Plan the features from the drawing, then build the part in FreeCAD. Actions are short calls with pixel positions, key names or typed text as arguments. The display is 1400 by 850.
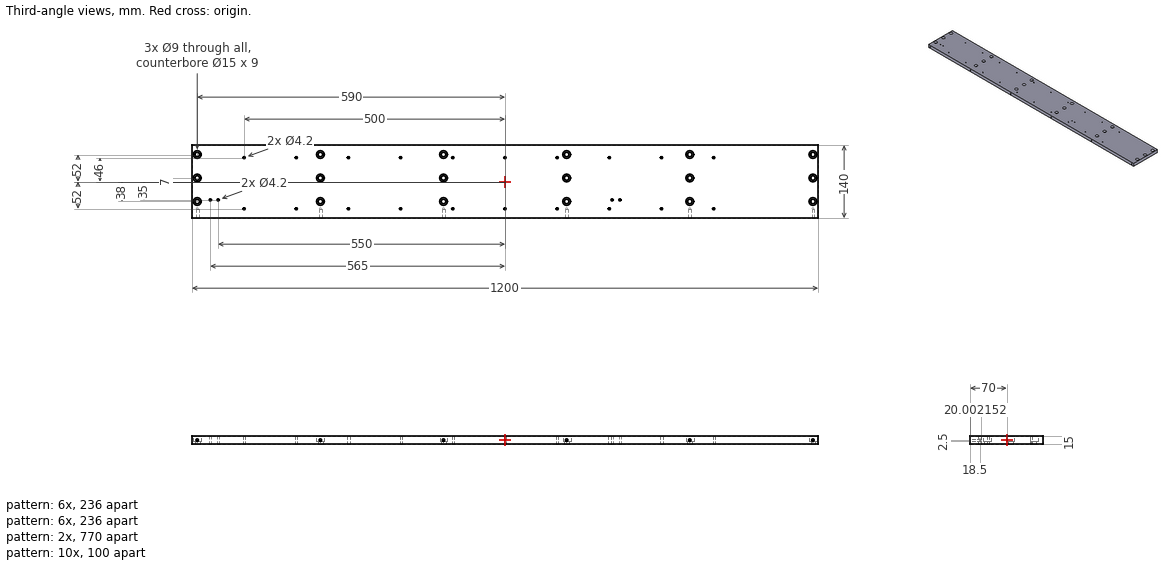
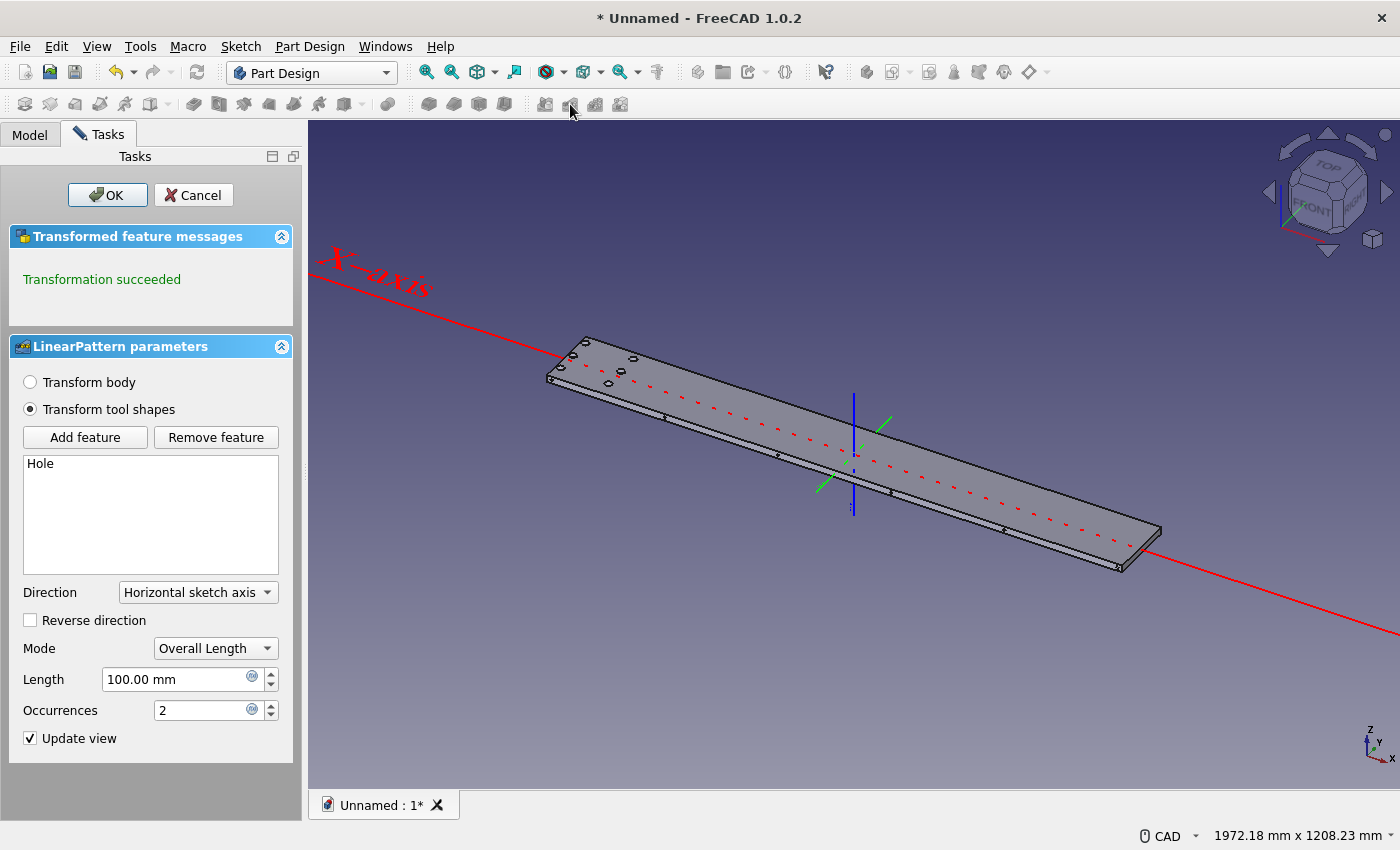
click(199, 592)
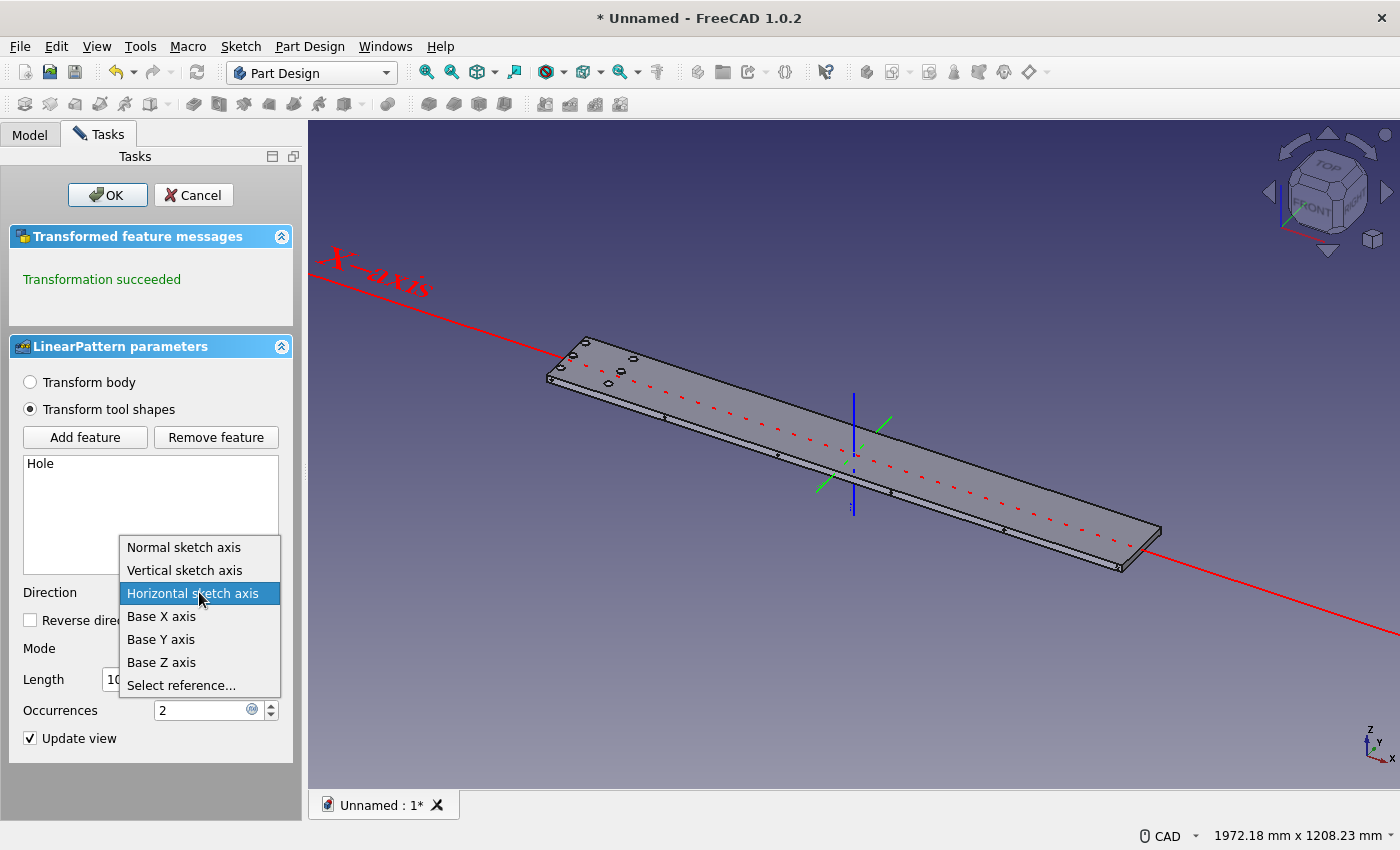
click(198, 616)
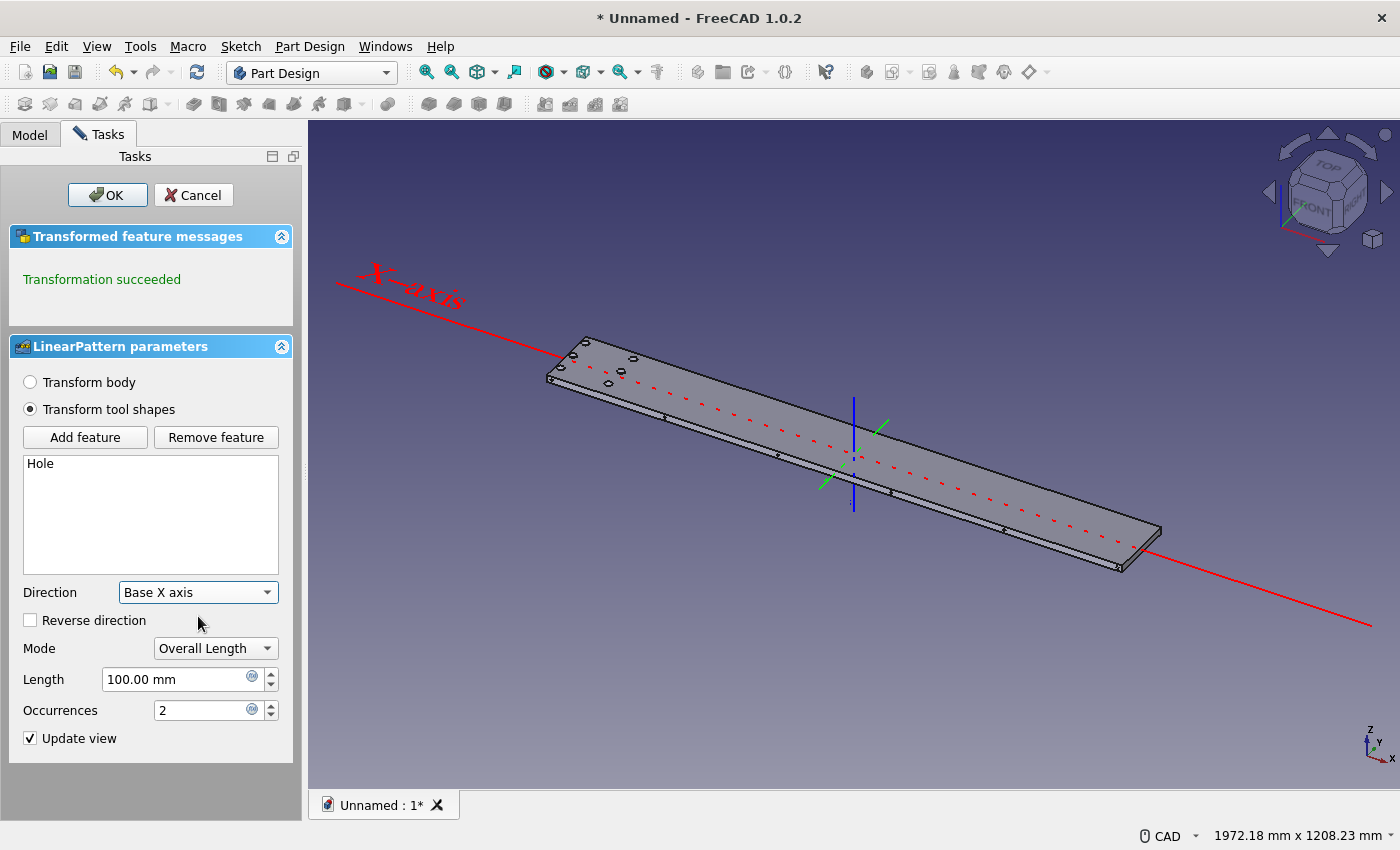
click(216, 648)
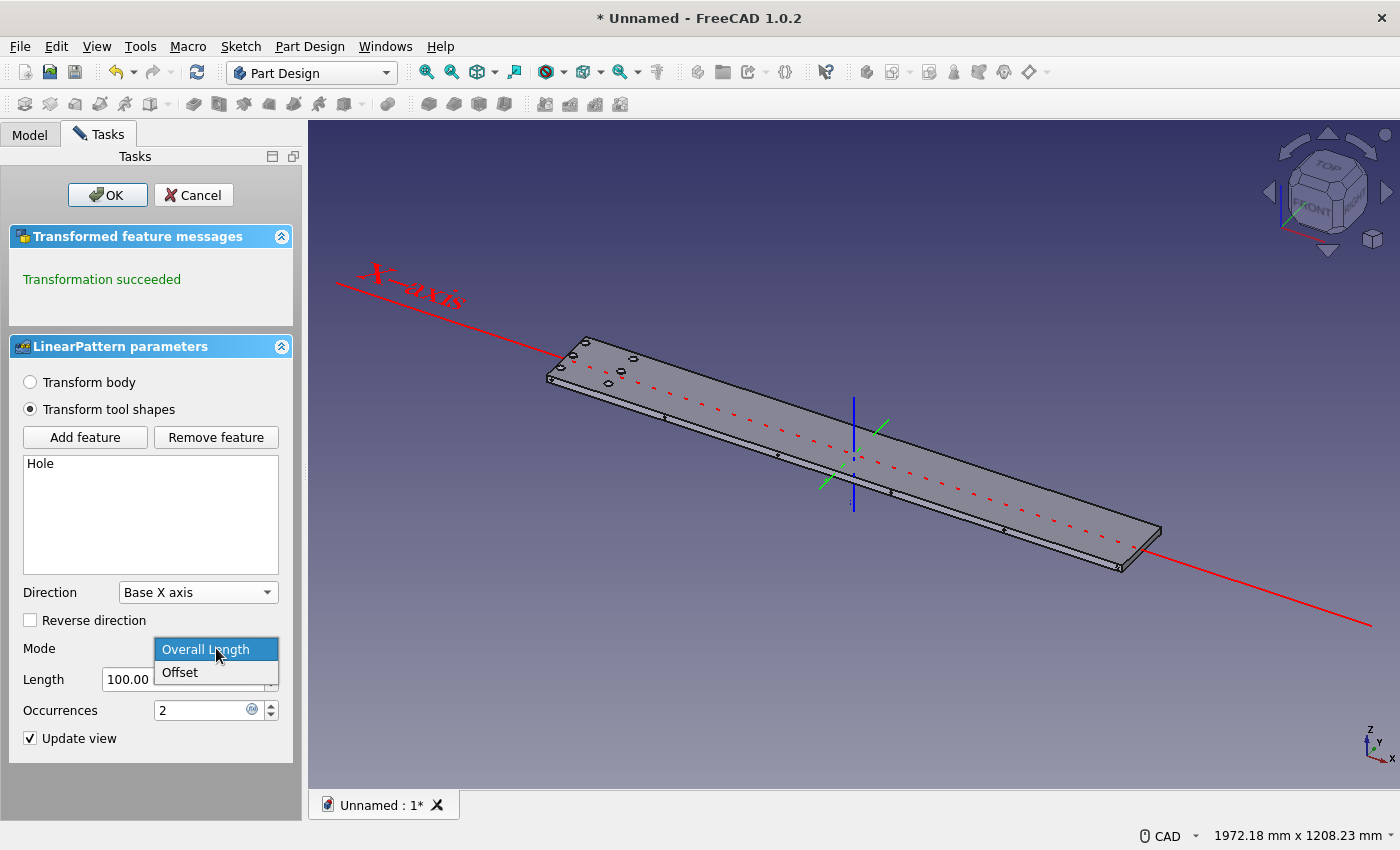
click(214, 672)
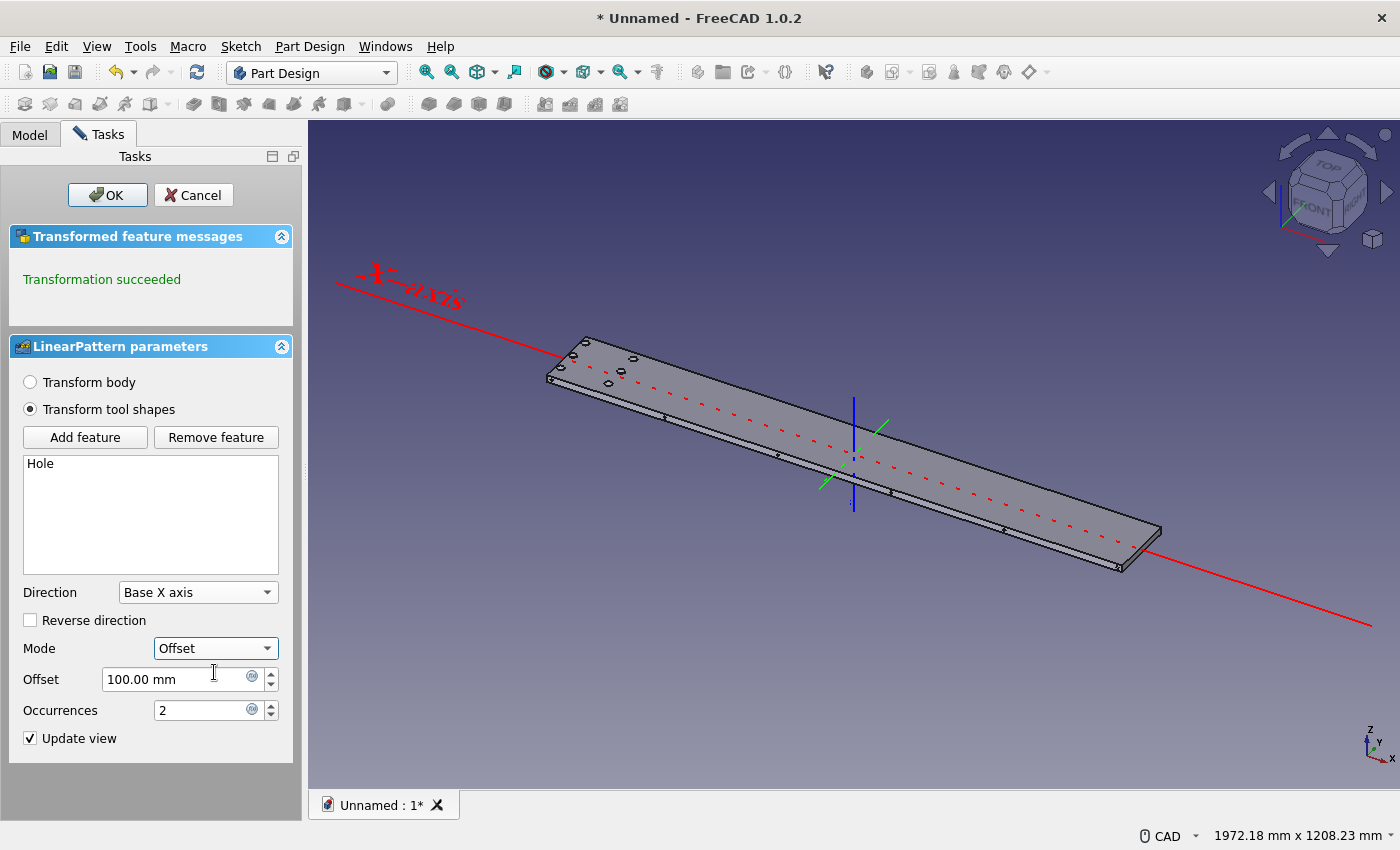
triple_click(184, 680)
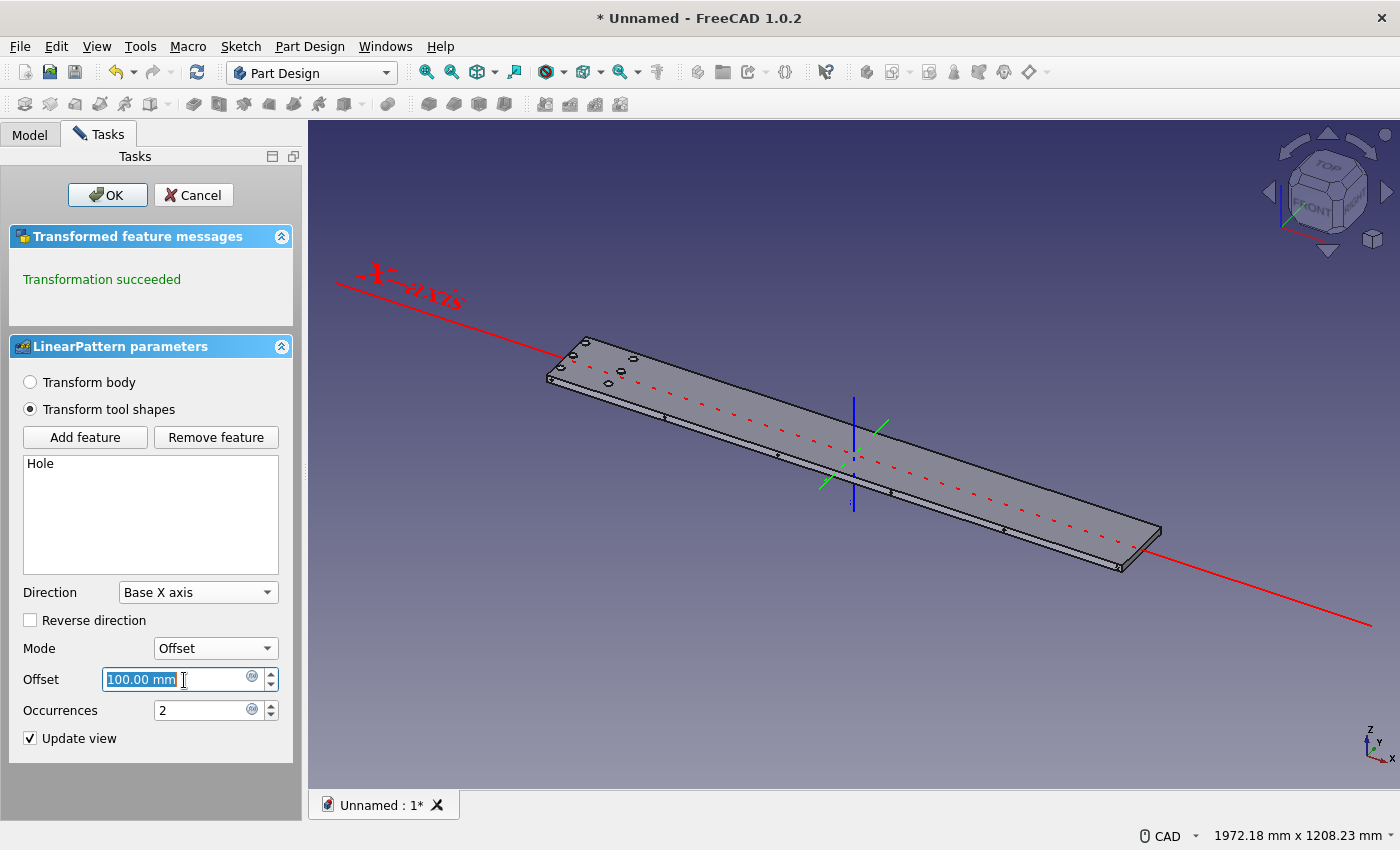
text(236)
key(Tab)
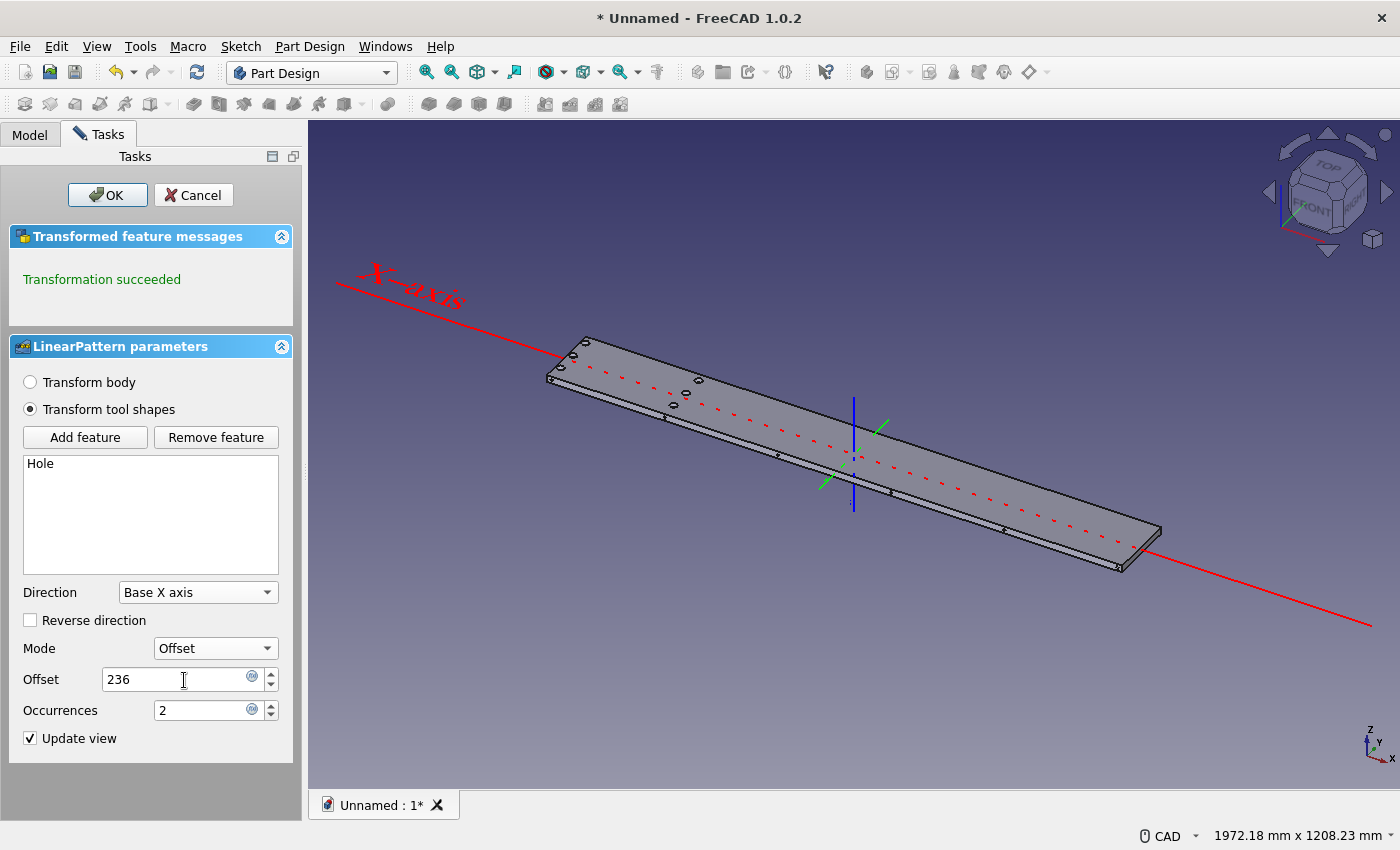
triple_click(210, 710)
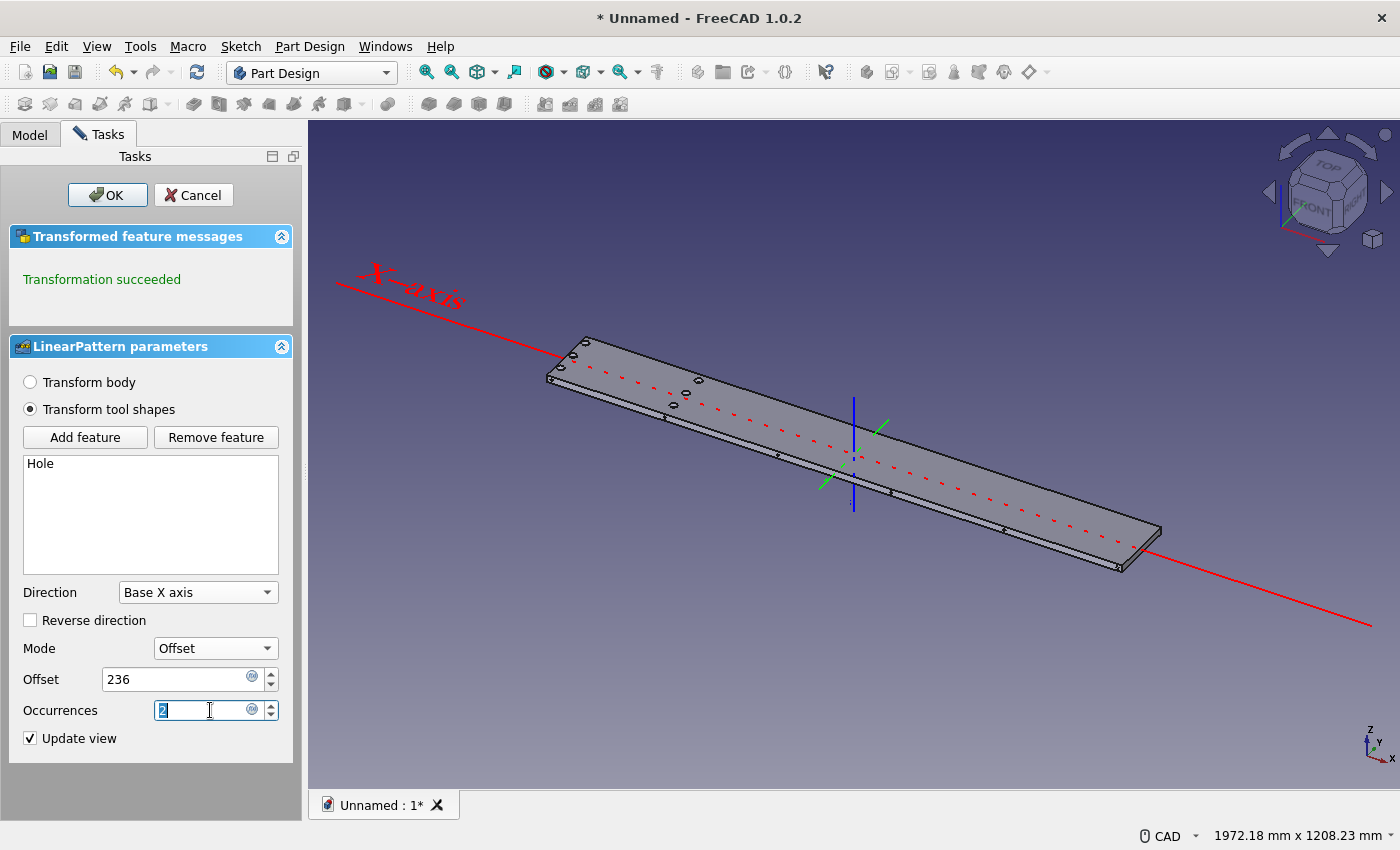
text(6)
key(Tab)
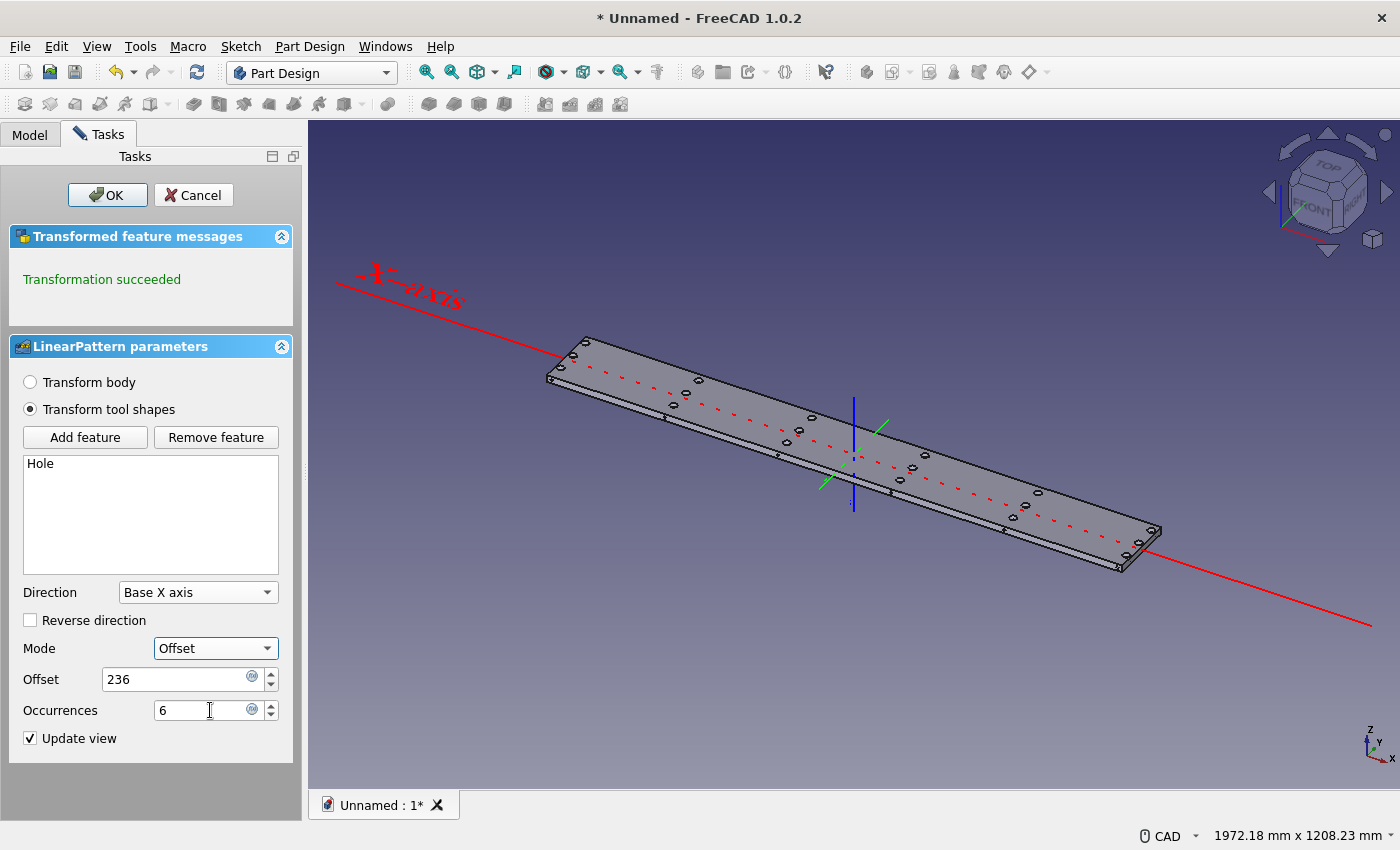
click(108, 195)